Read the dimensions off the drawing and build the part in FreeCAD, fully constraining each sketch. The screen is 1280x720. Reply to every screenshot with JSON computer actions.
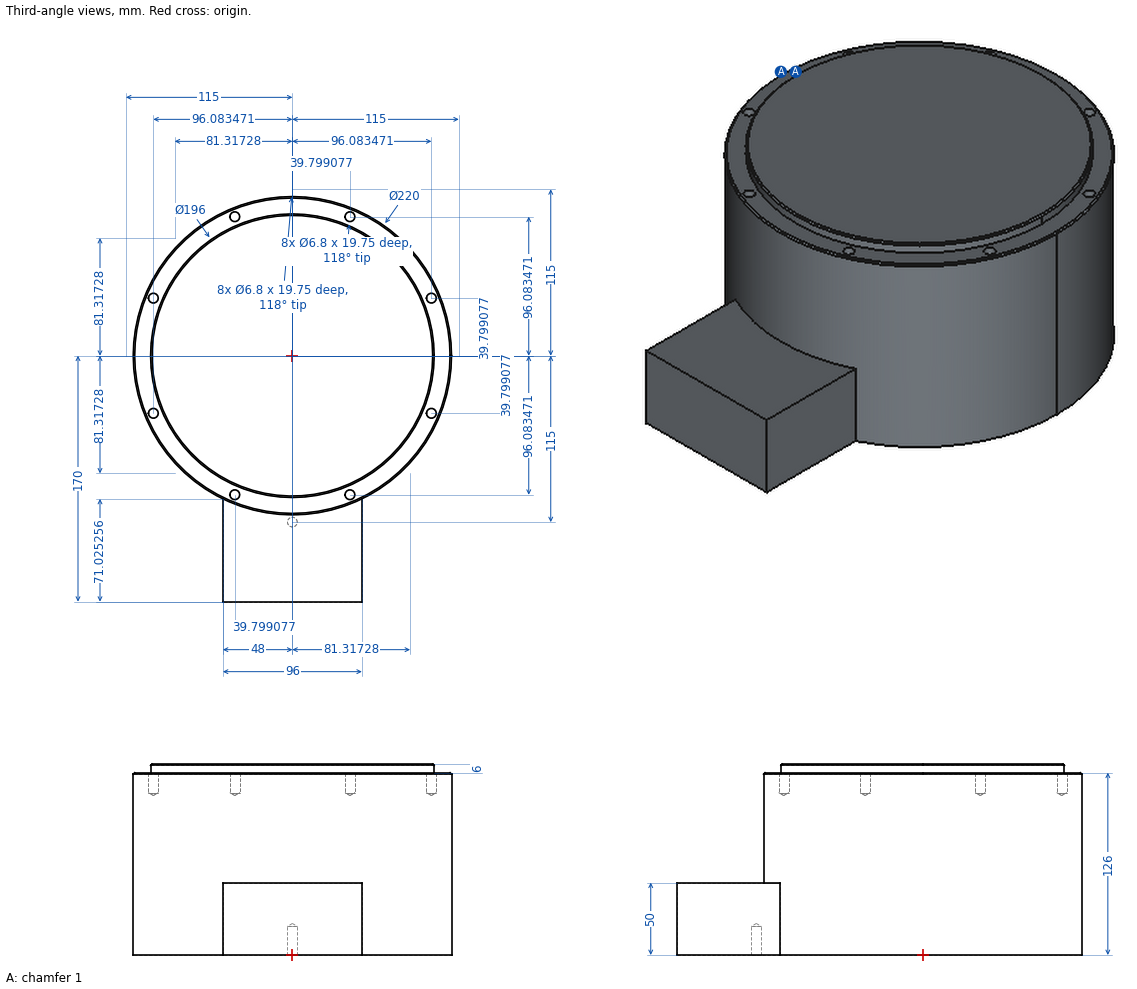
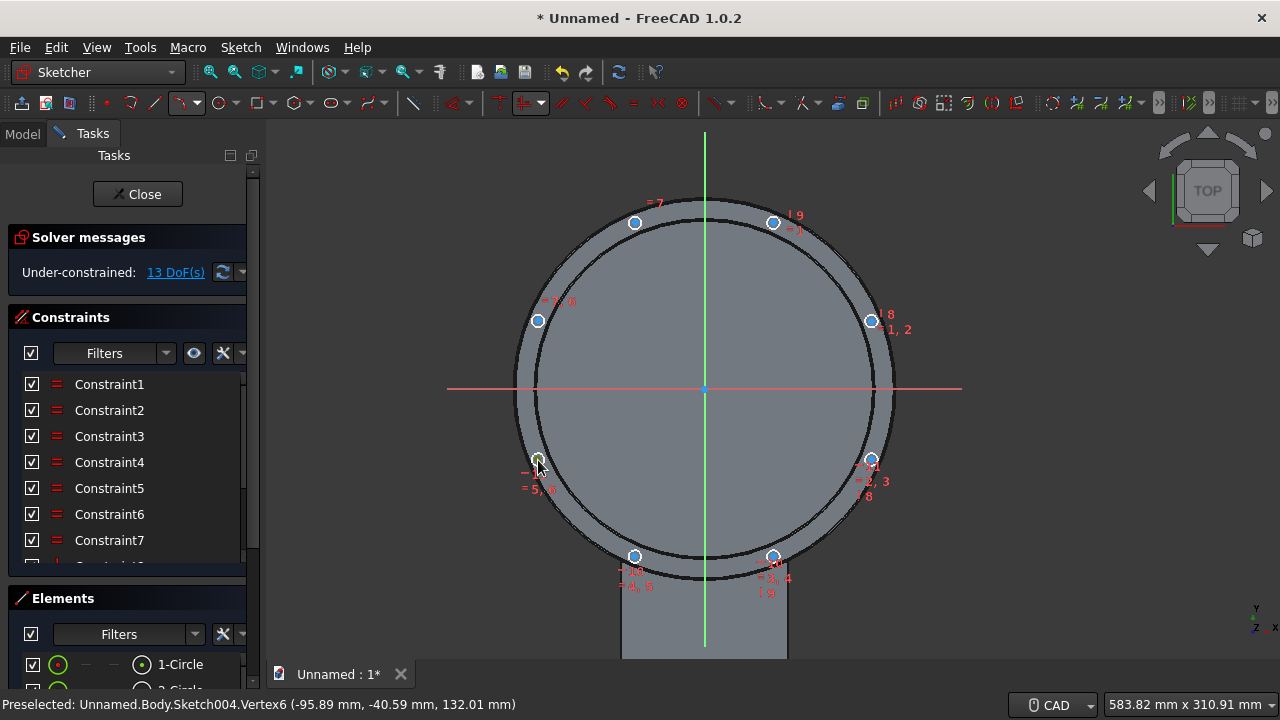
{"action": "left_click", "coordinate": [538, 321]}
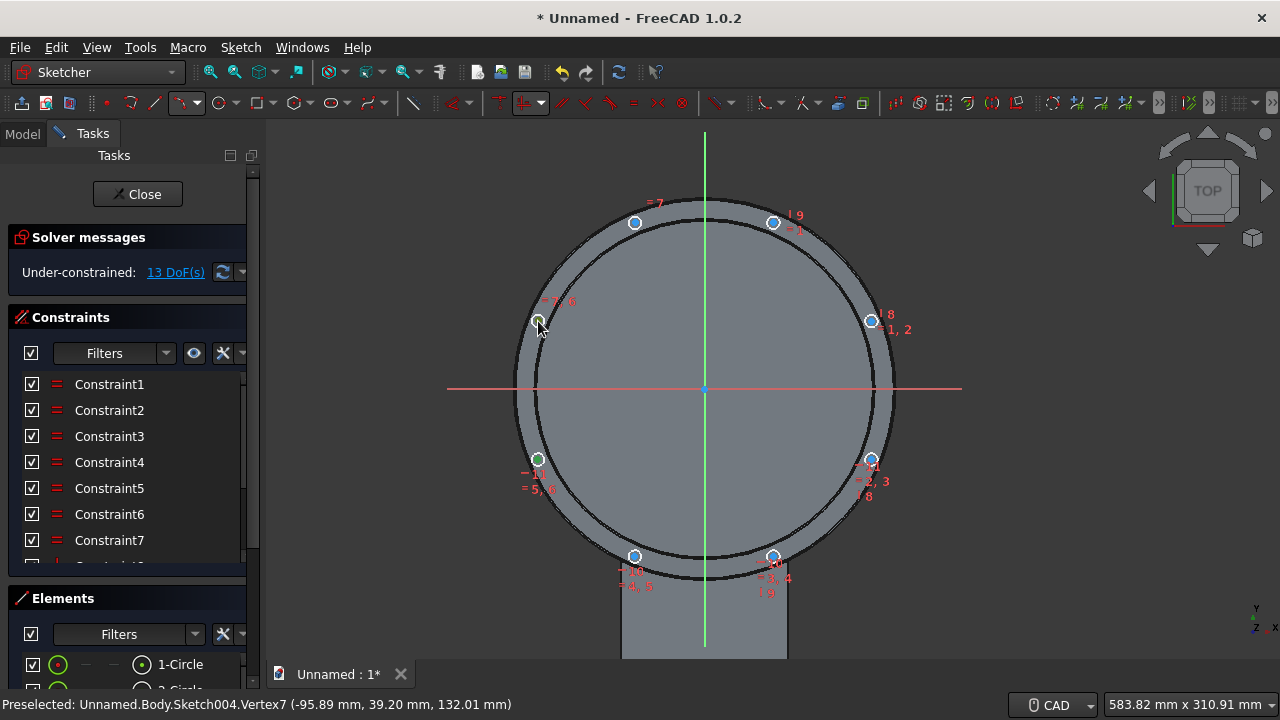
{"action": "key", "text": "v"}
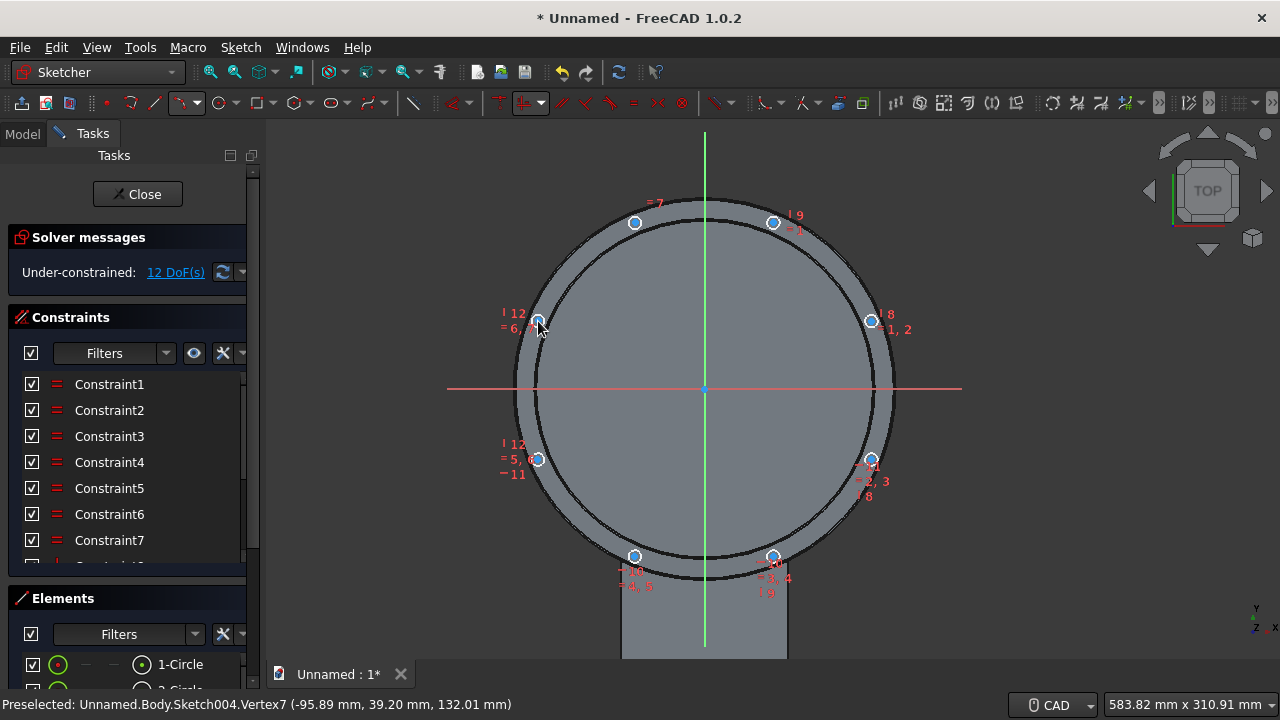
{"action": "left_click", "coordinate": [871, 321]}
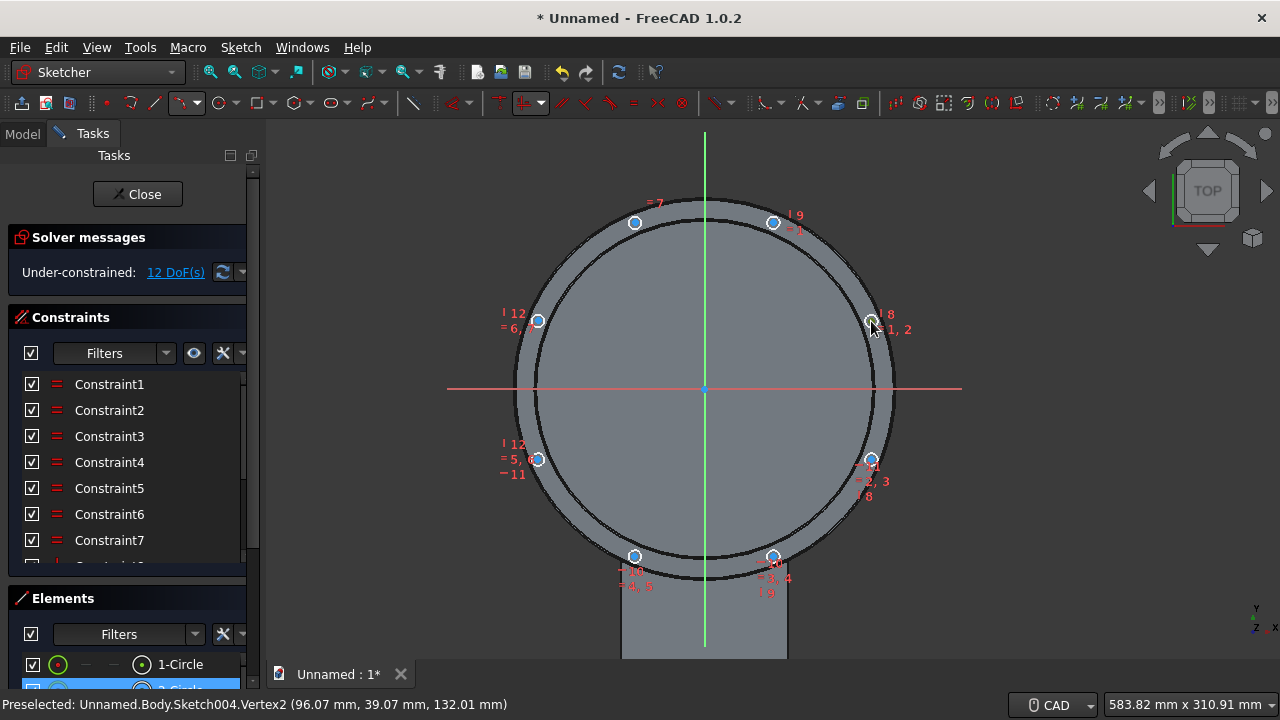
{"action": "left_click", "coordinate": [538, 321]}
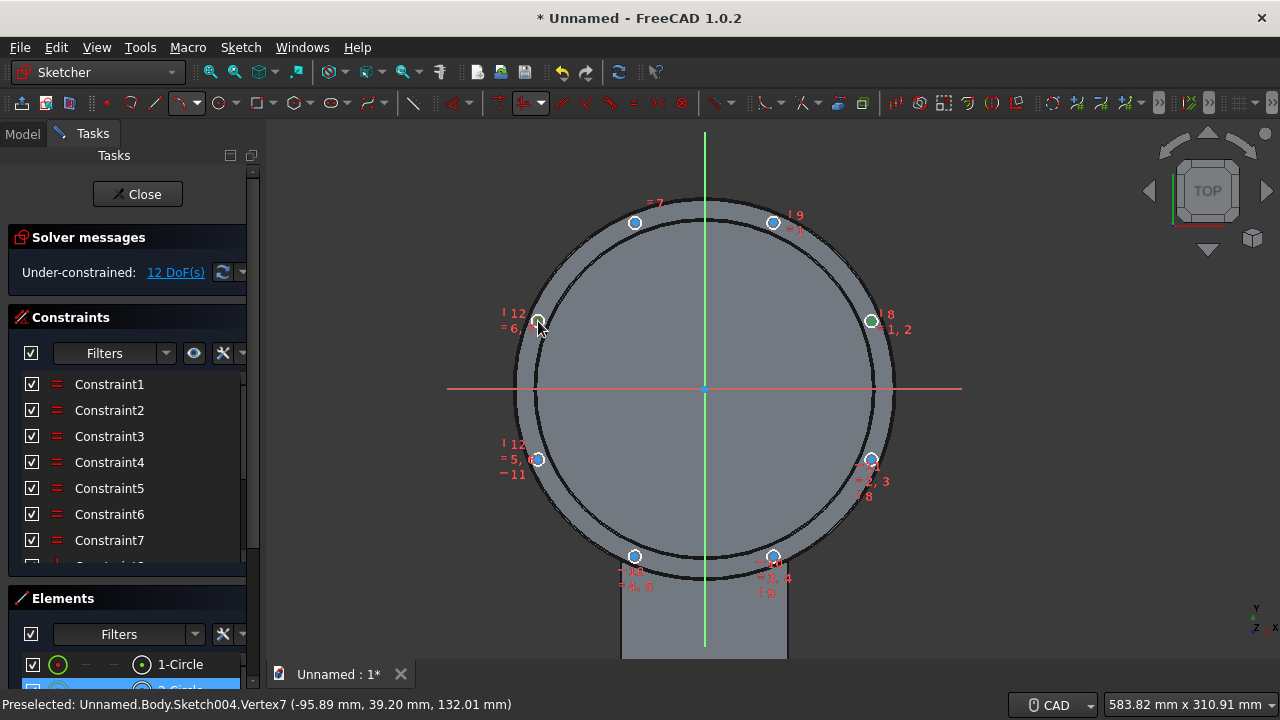
{"action": "left_click", "coordinate": [544, 104]}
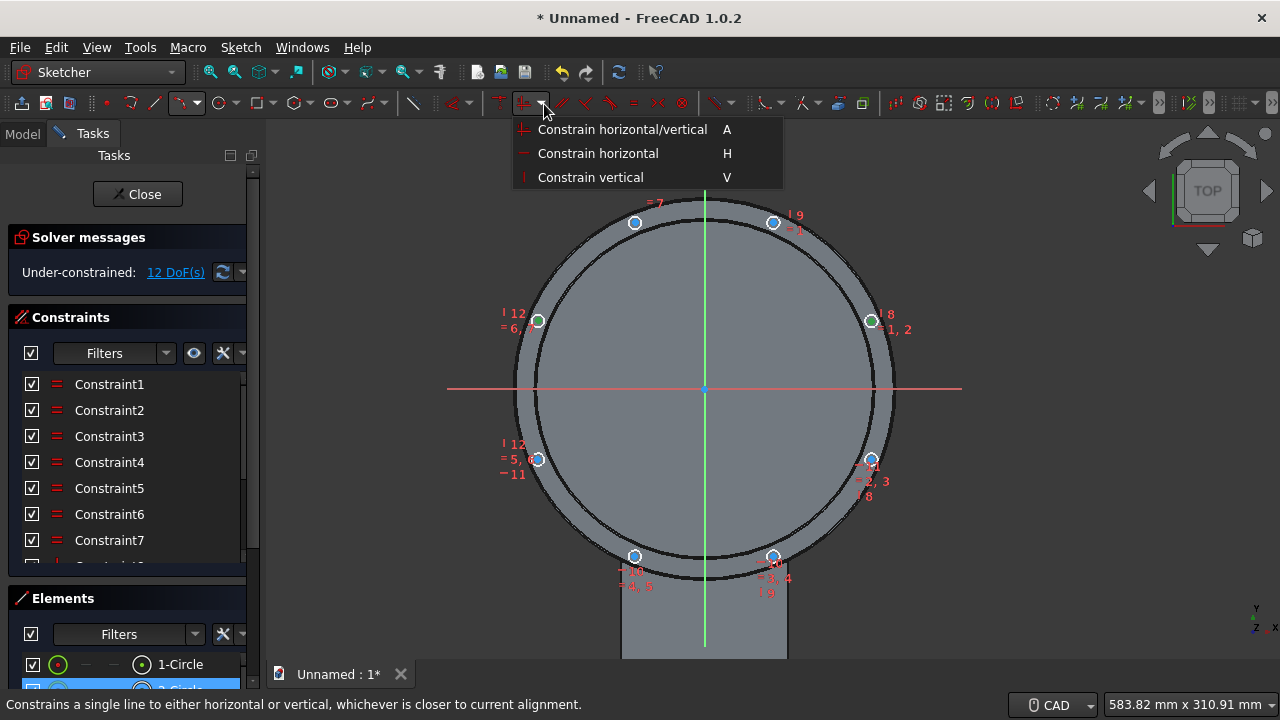
{"action": "left_click", "coordinate": [648, 153]}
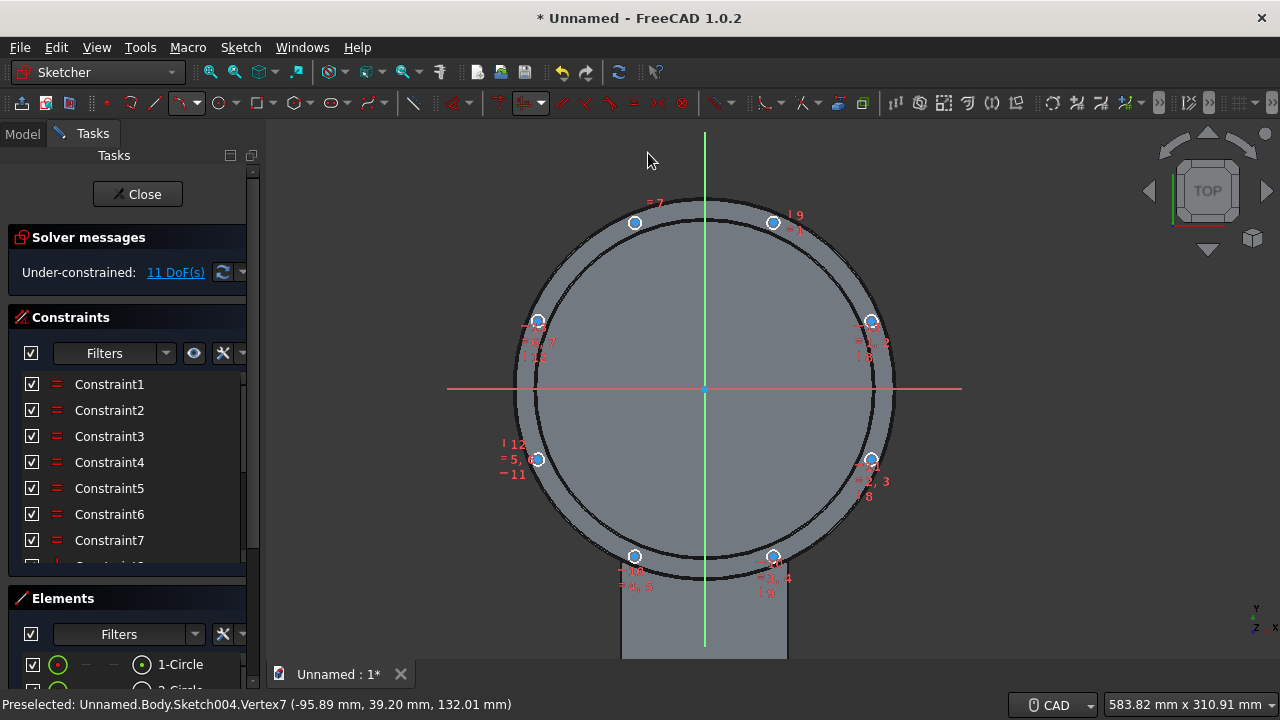
{"action": "left_click", "coordinate": [635, 557]}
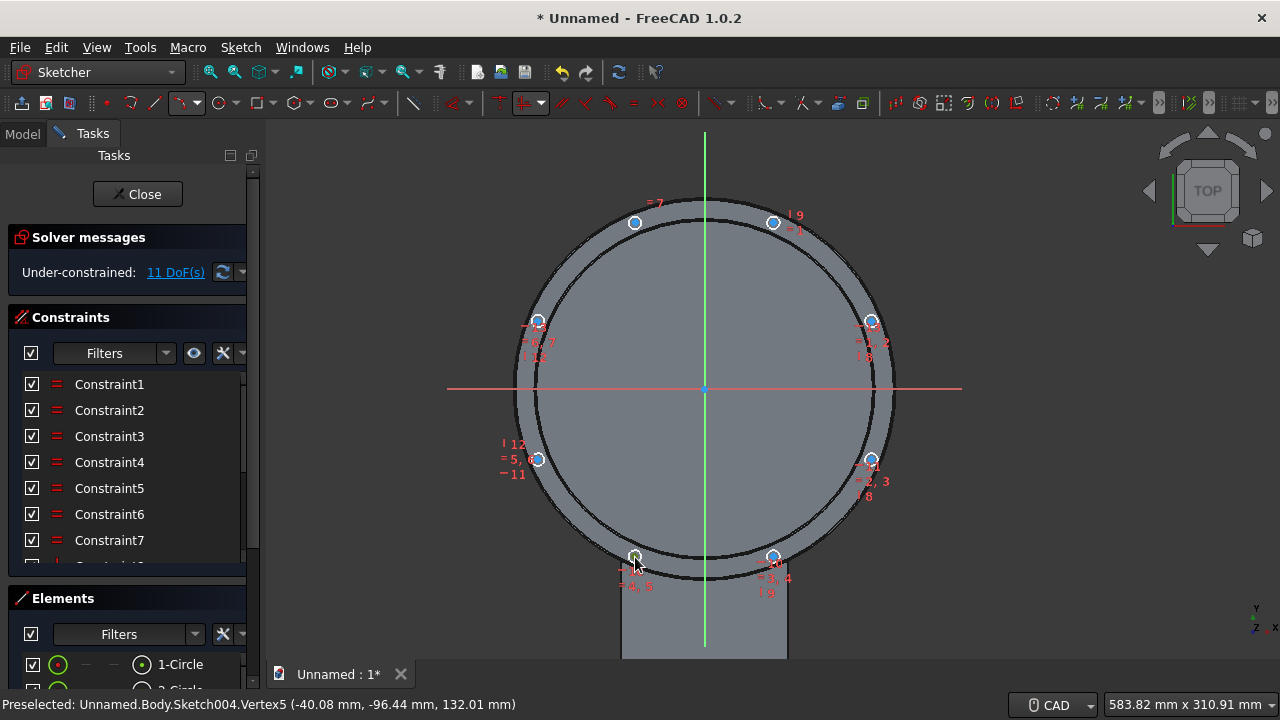
{"action": "left_click", "coordinate": [635, 223]}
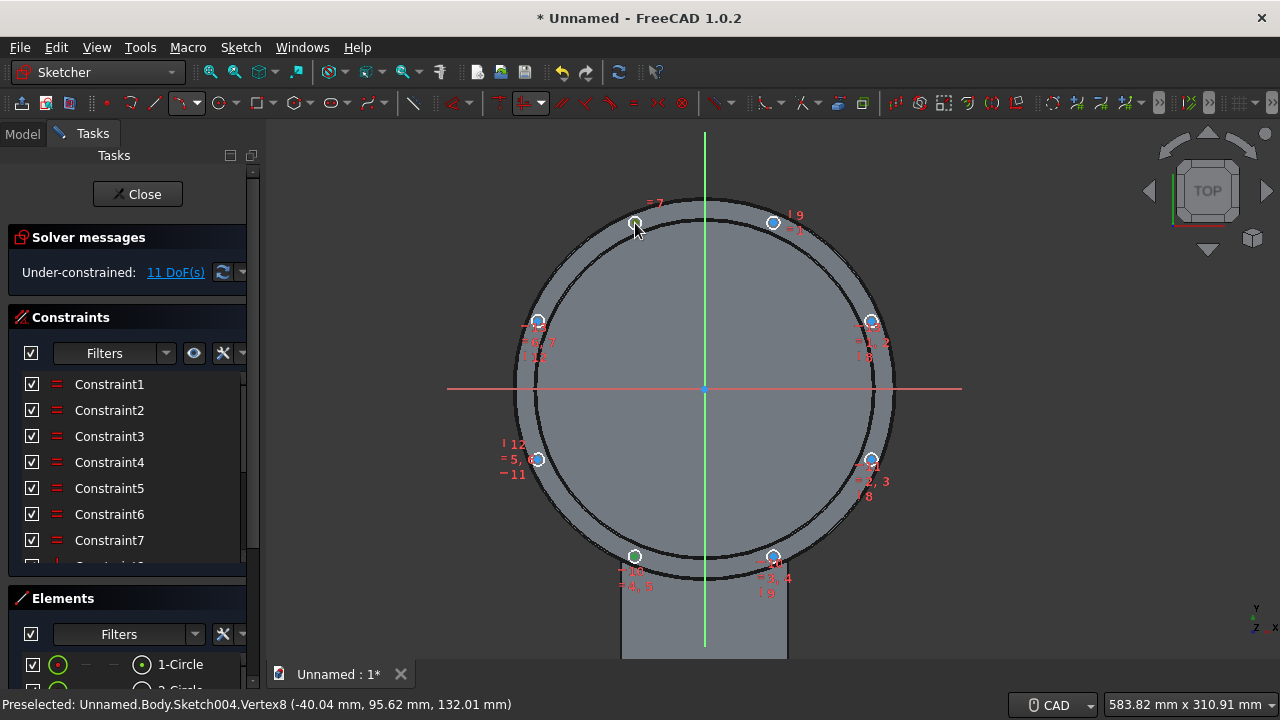
{"action": "key", "text": "v"}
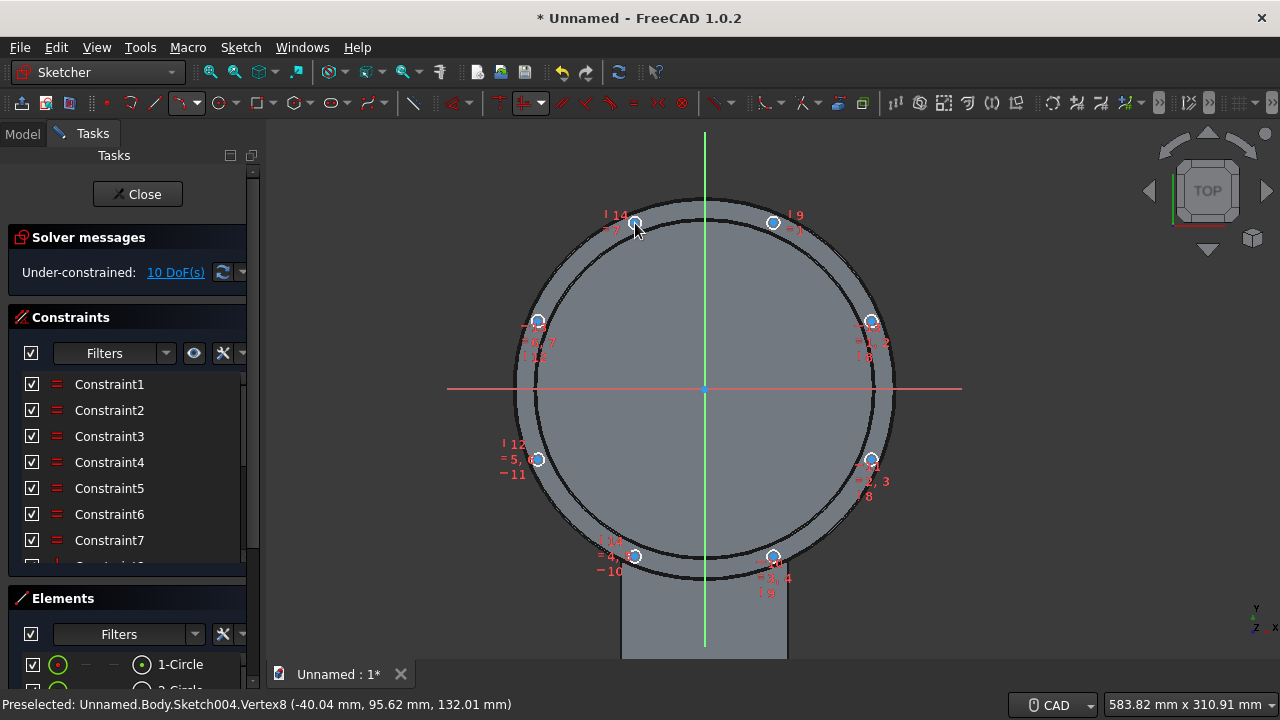
{"action": "left_click", "coordinate": [773, 223]}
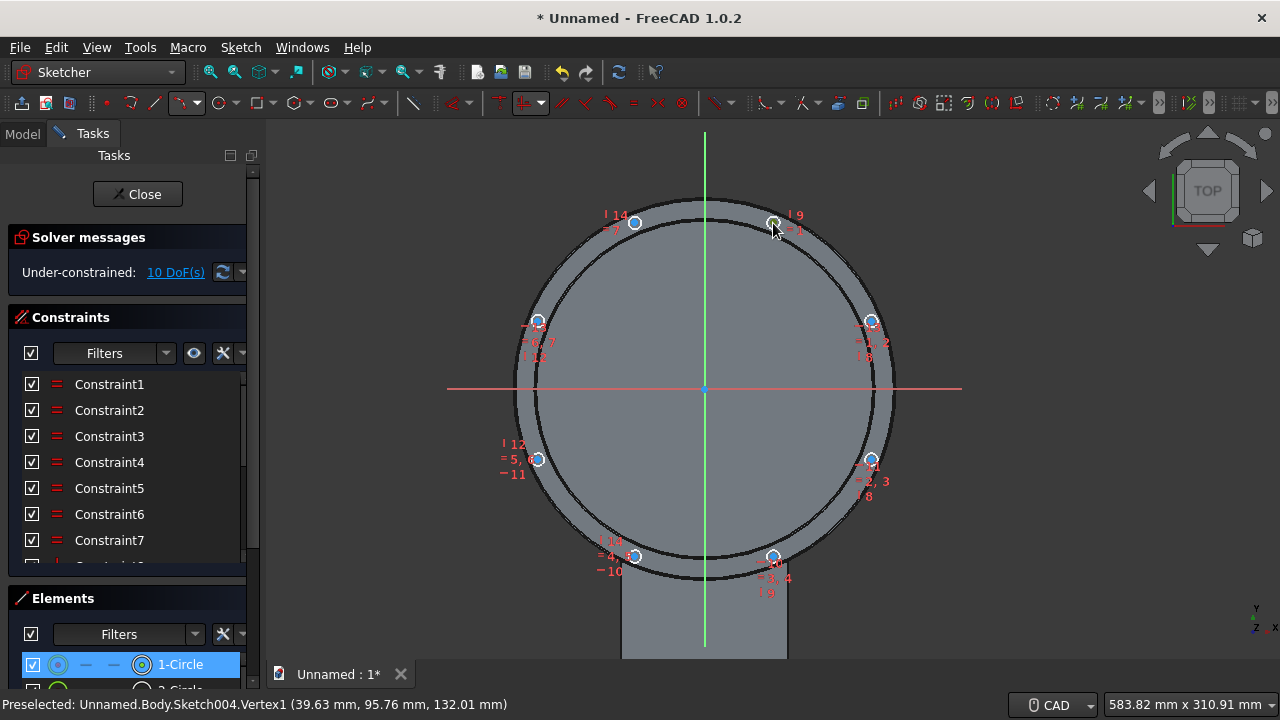
{"action": "left_click", "coordinate": [635, 223]}